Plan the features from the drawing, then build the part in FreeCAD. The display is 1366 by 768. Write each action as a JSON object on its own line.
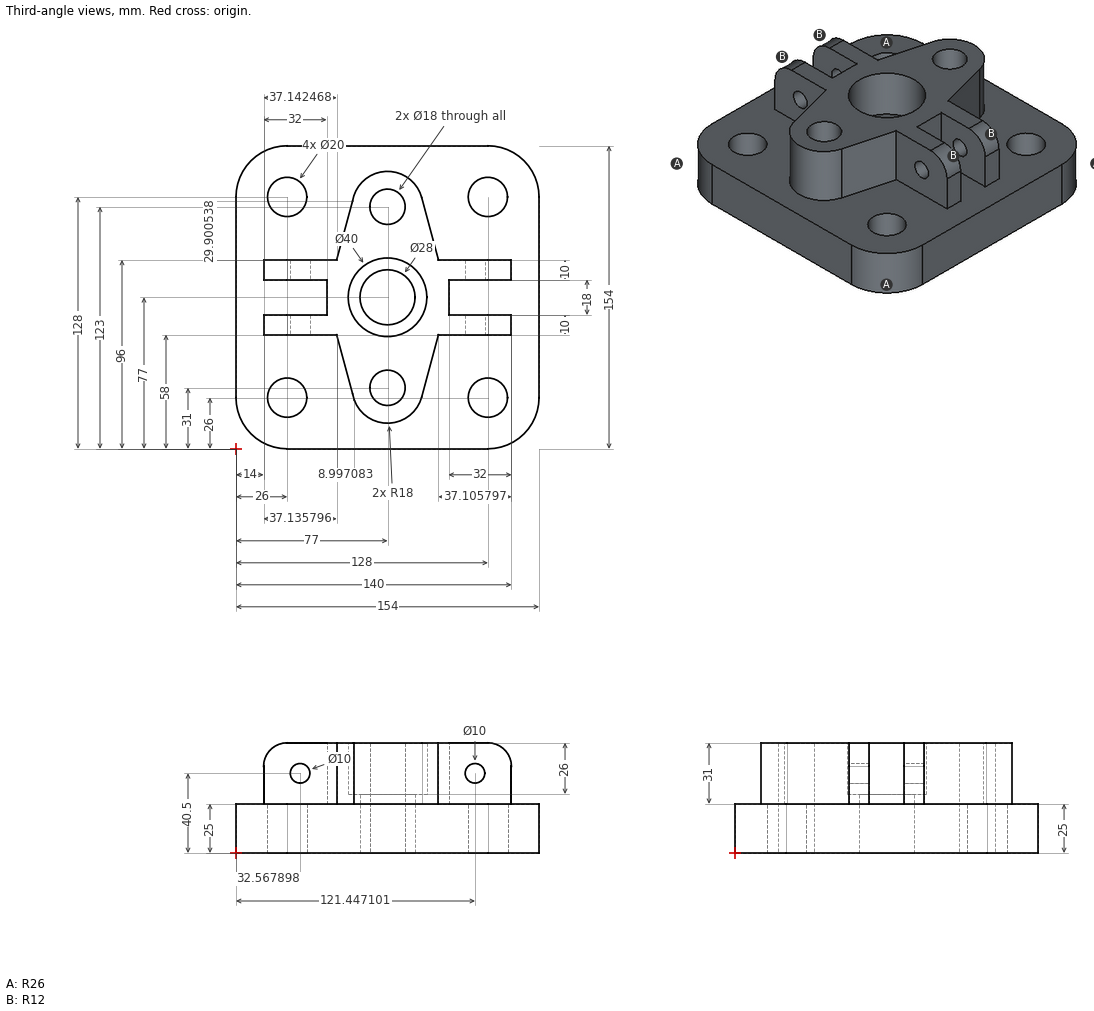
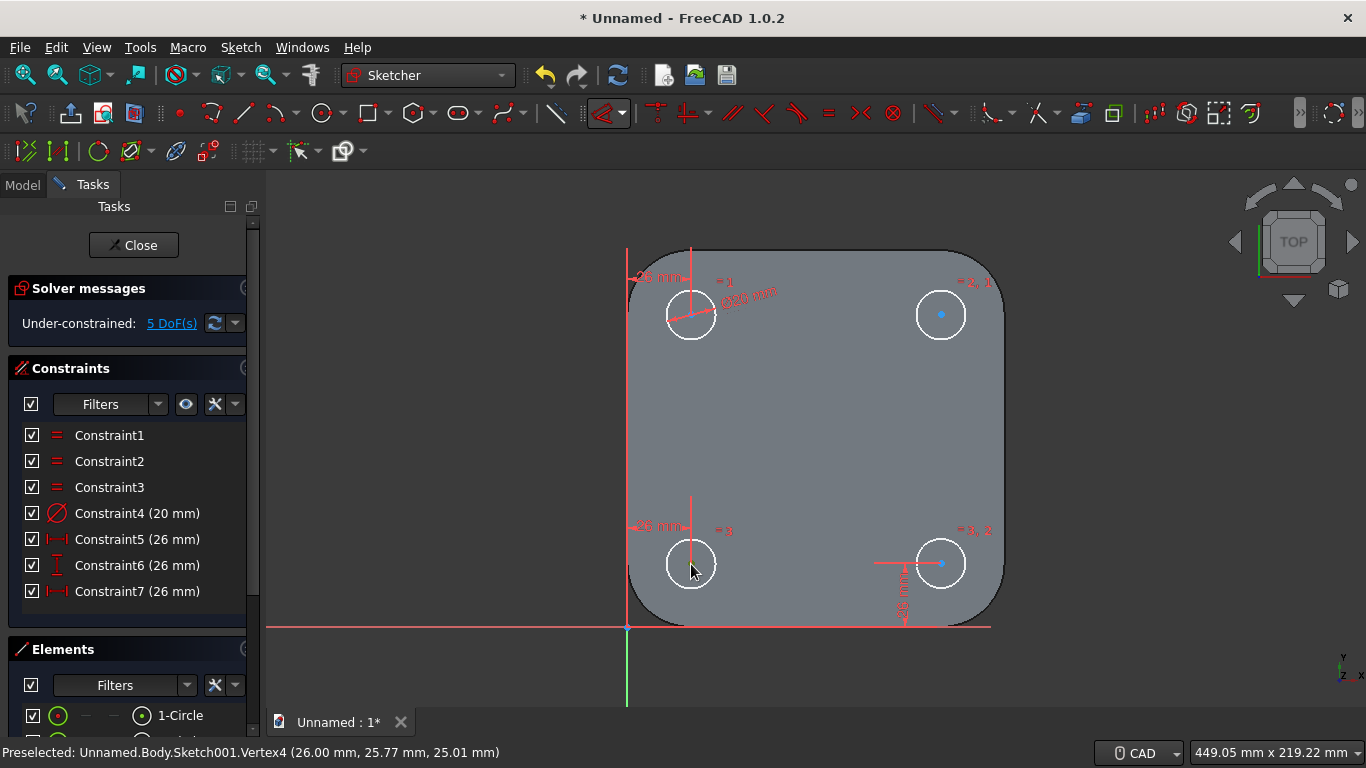
{"action": "key", "text": "i"}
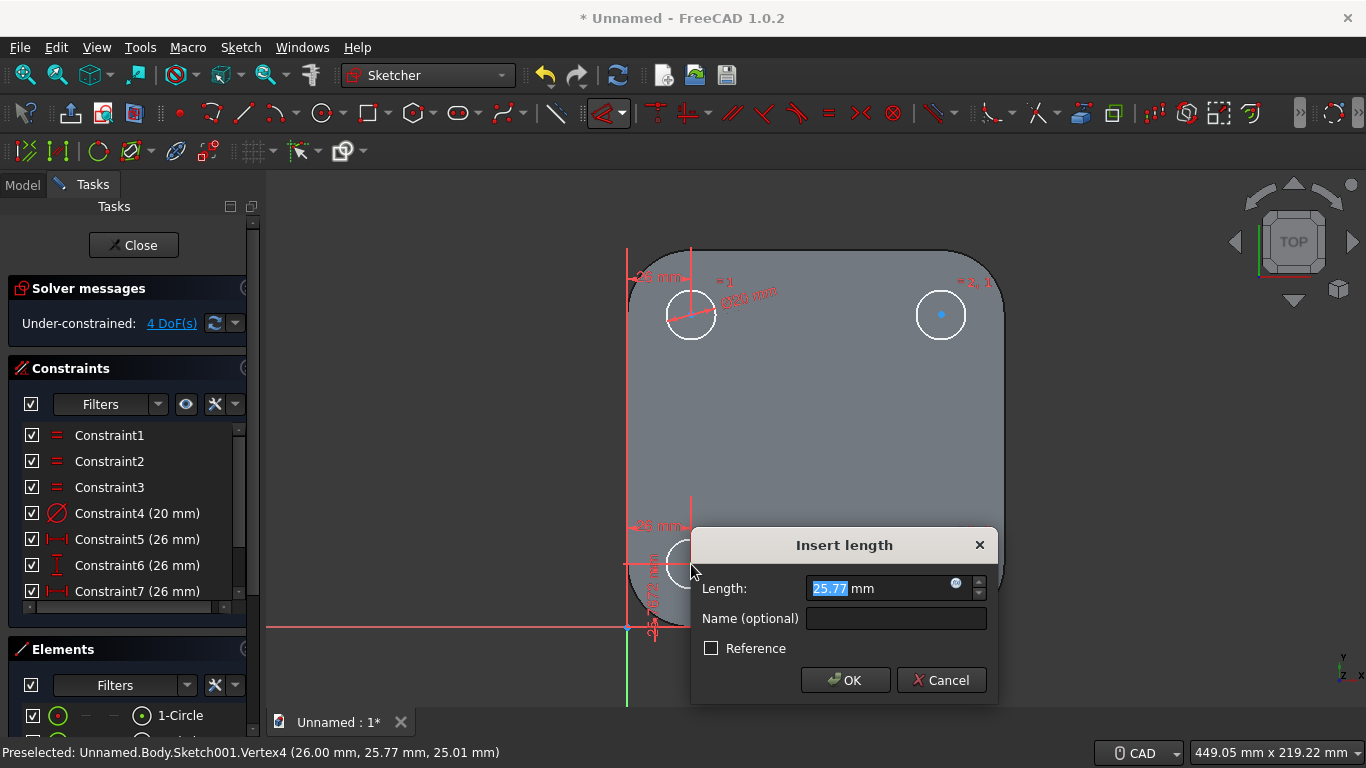
{"action": "type", "text": "26"}
{"action": "key", "text": "Return"}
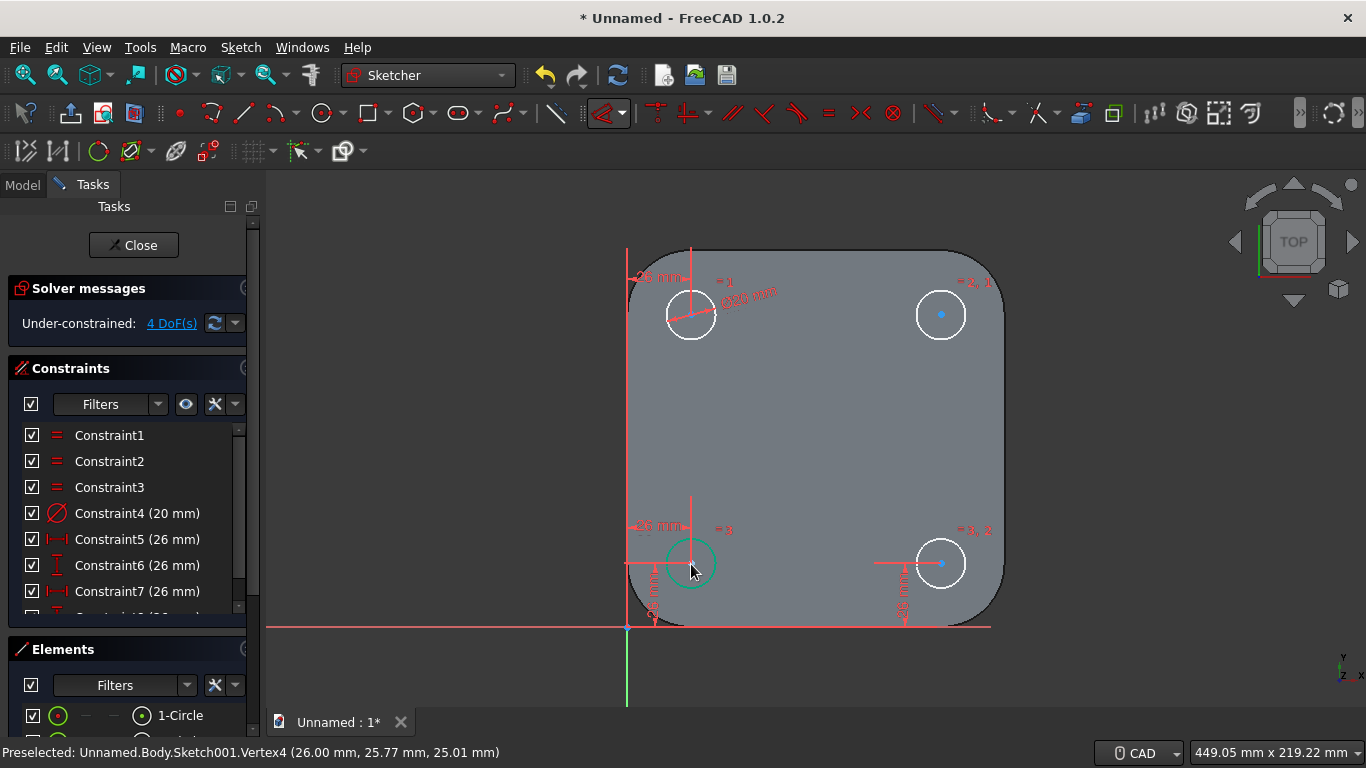
{"action": "left_click", "coordinate": [691, 315]}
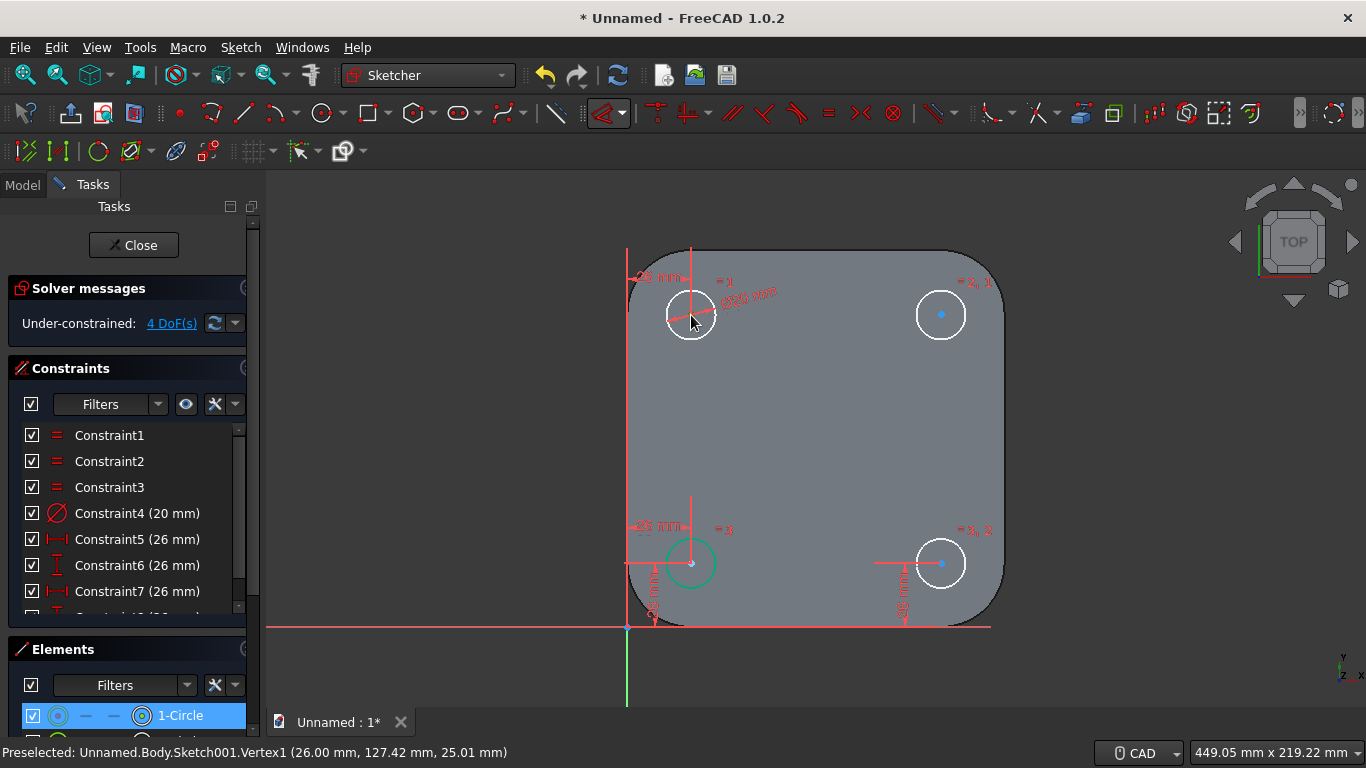
{"action": "left_click", "coordinate": [624, 114]}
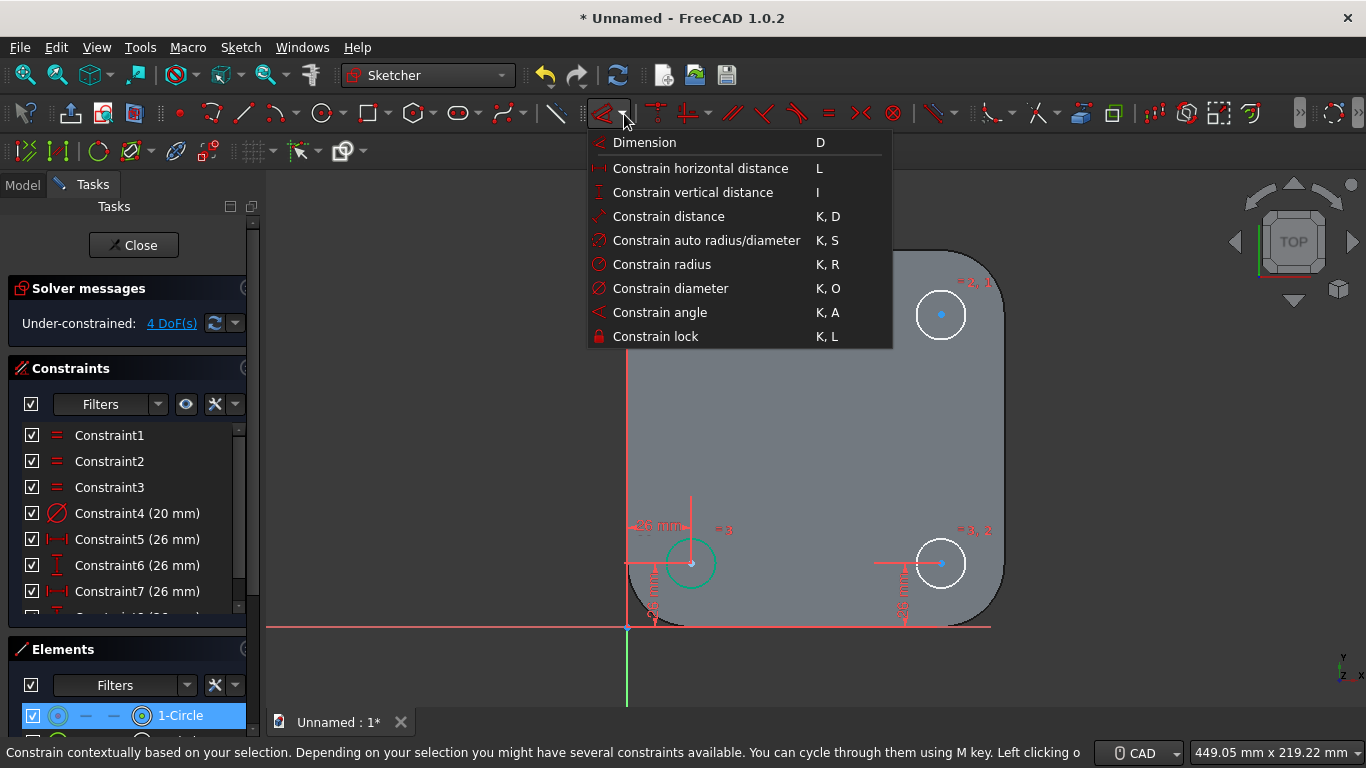
{"action": "left_click", "coordinate": [740, 192]}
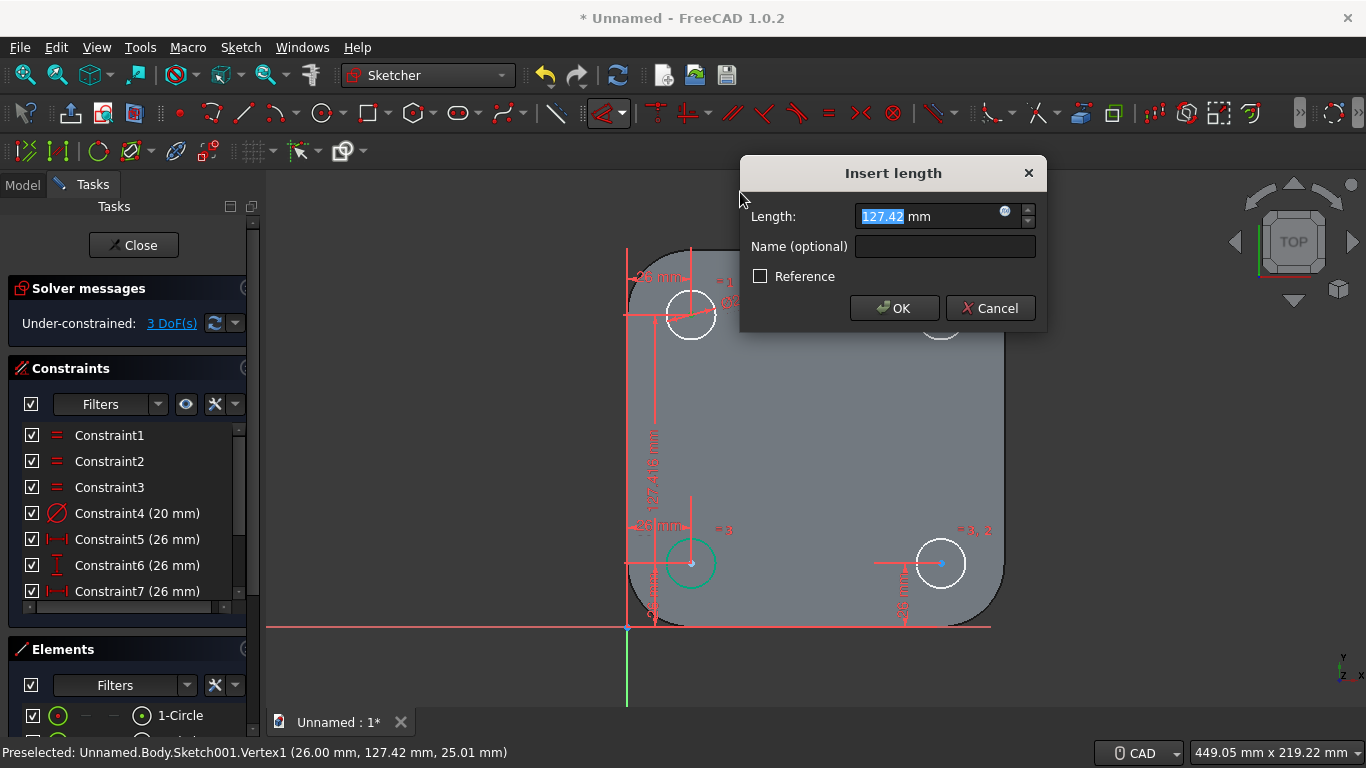
{"action": "type", "text": "128"}
{"action": "key", "text": "Return"}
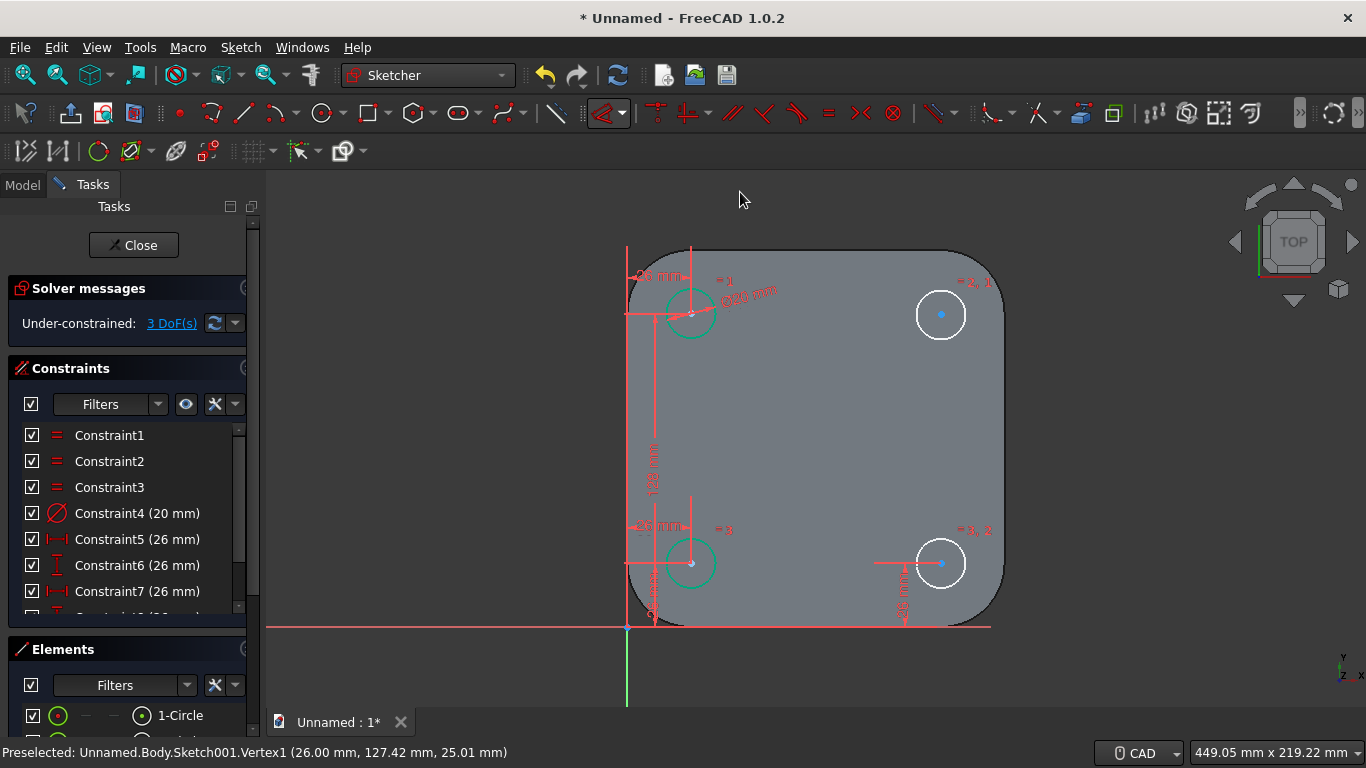
{"action": "left_click", "coordinate": [941, 315]}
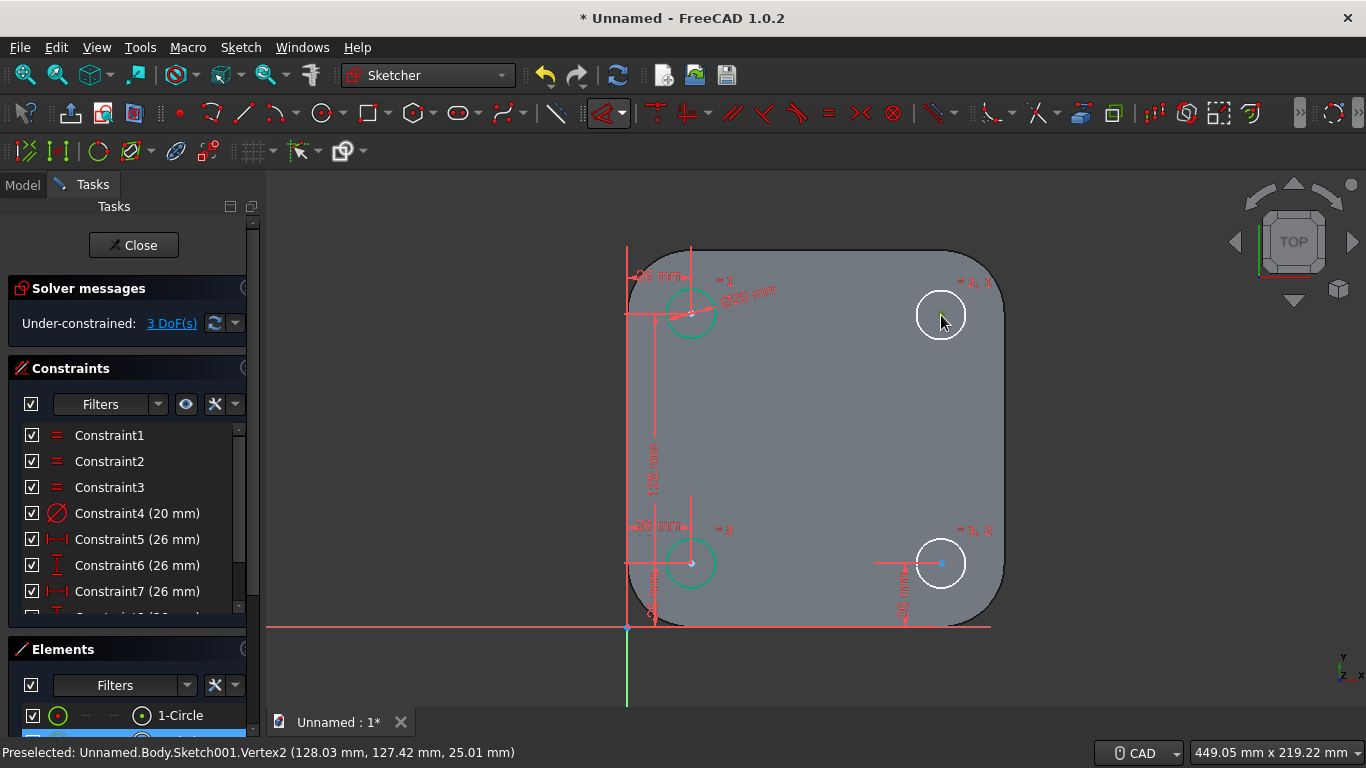
{"action": "left_click", "coordinate": [624, 114]}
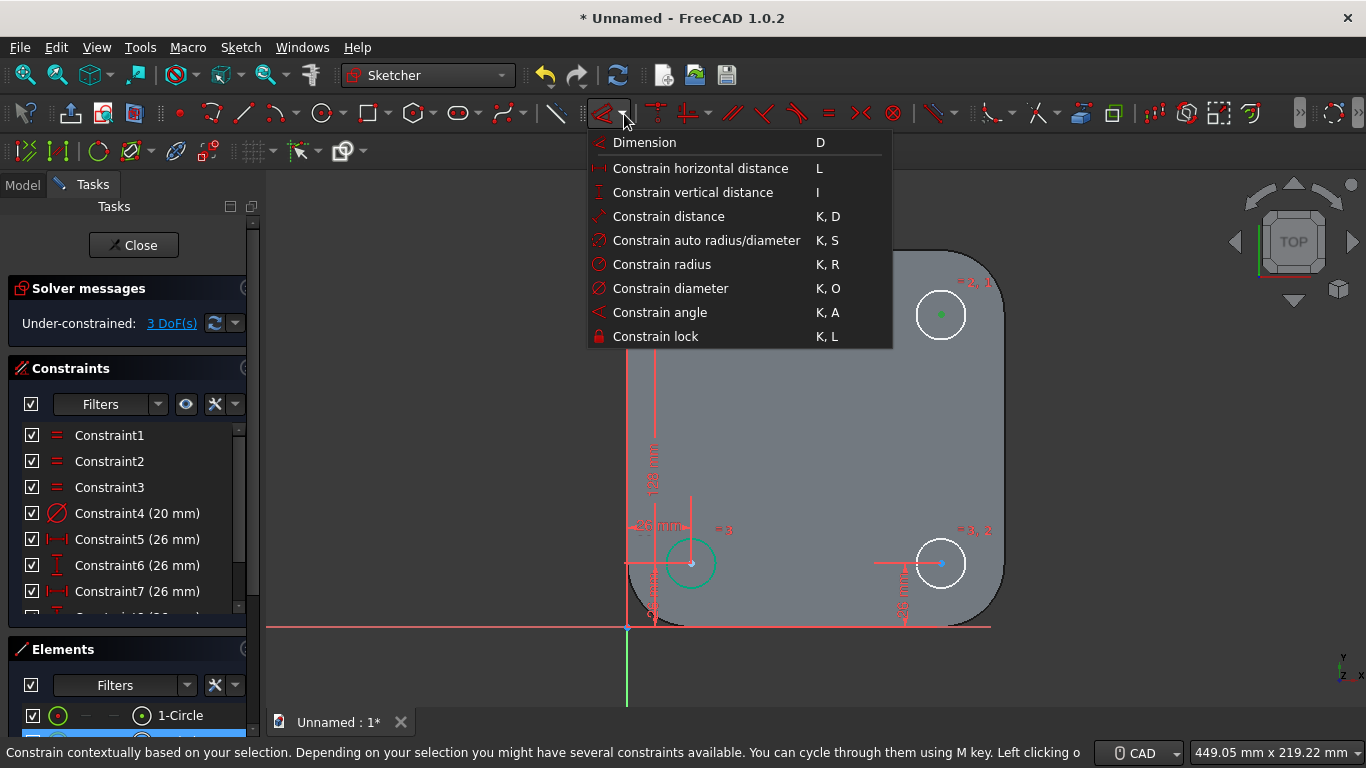
{"action": "left_click", "coordinate": [740, 168]}